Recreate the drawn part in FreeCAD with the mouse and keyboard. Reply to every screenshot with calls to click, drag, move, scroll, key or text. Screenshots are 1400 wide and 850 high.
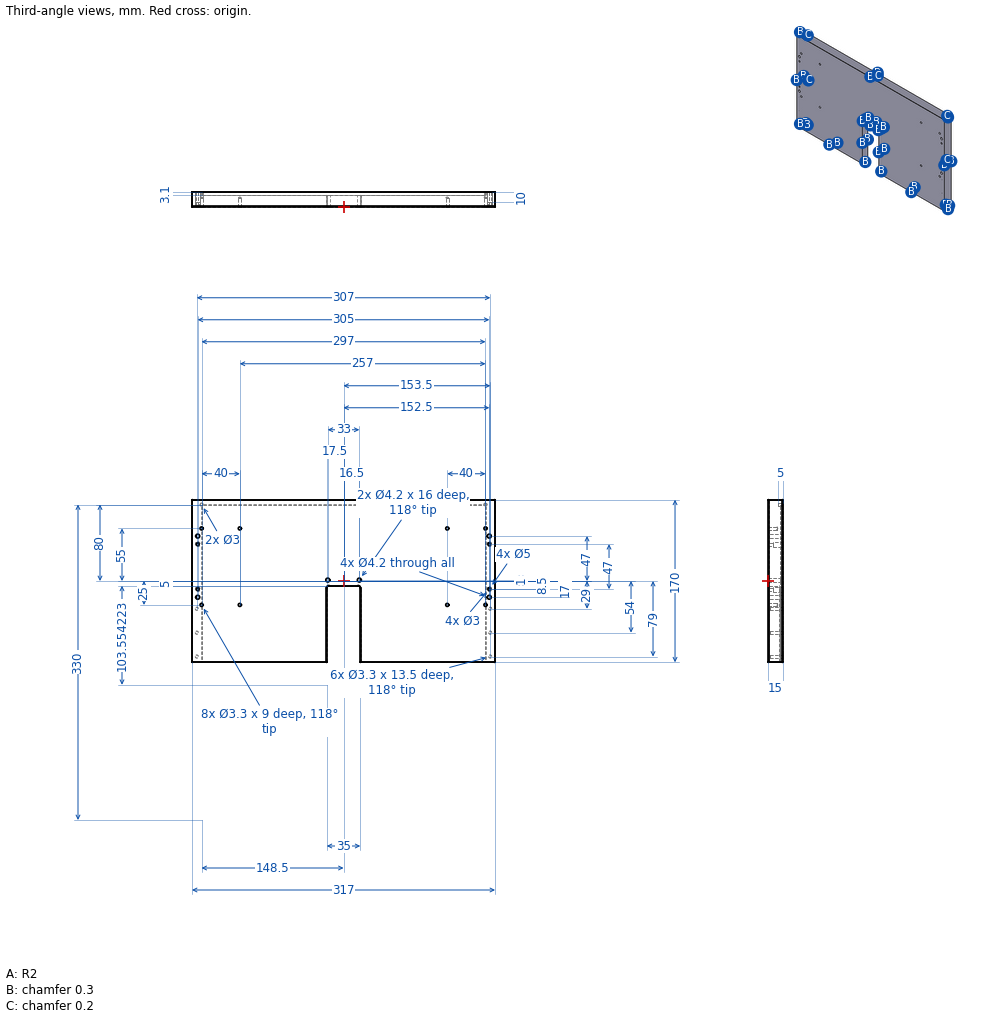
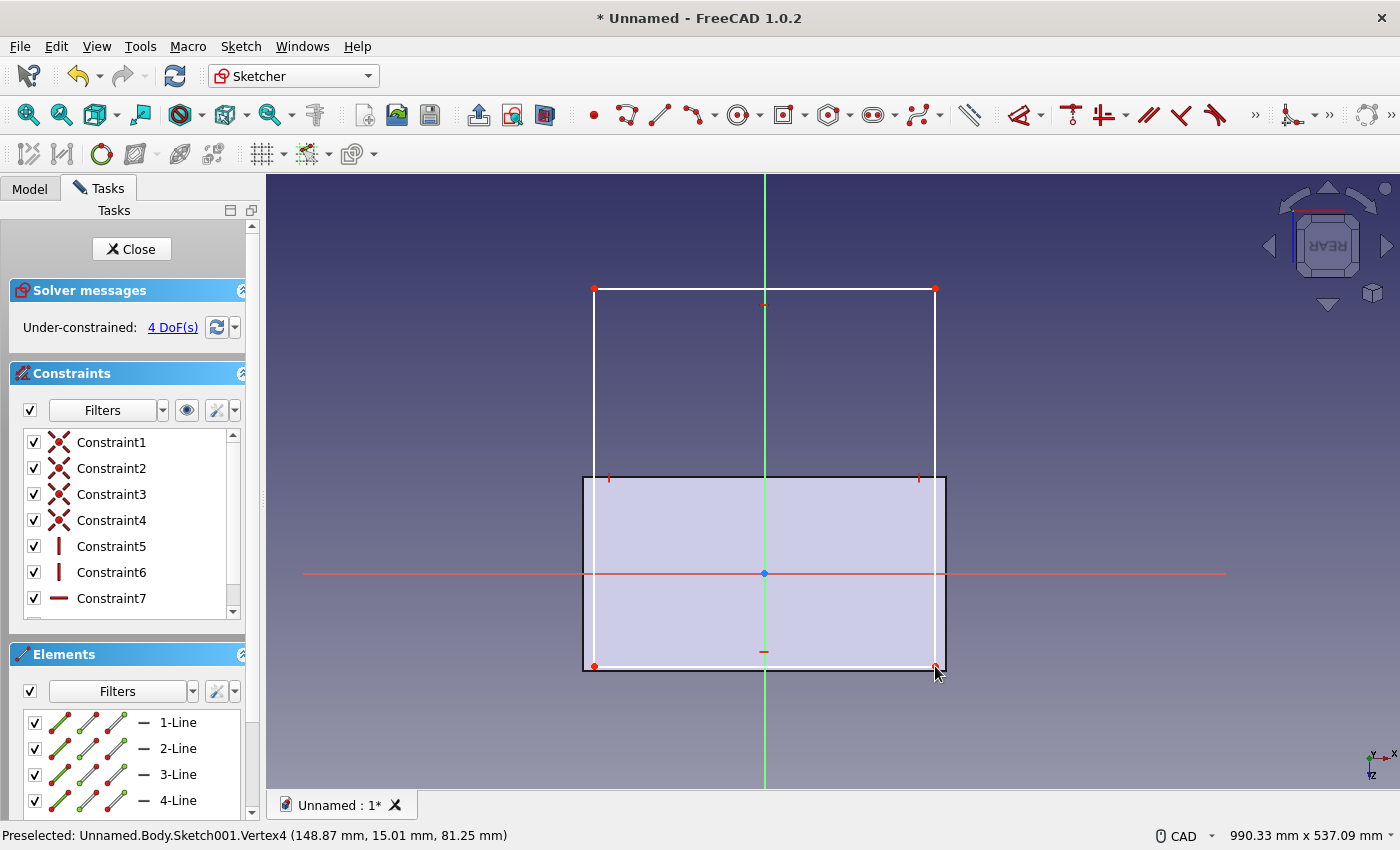
click(1018, 116)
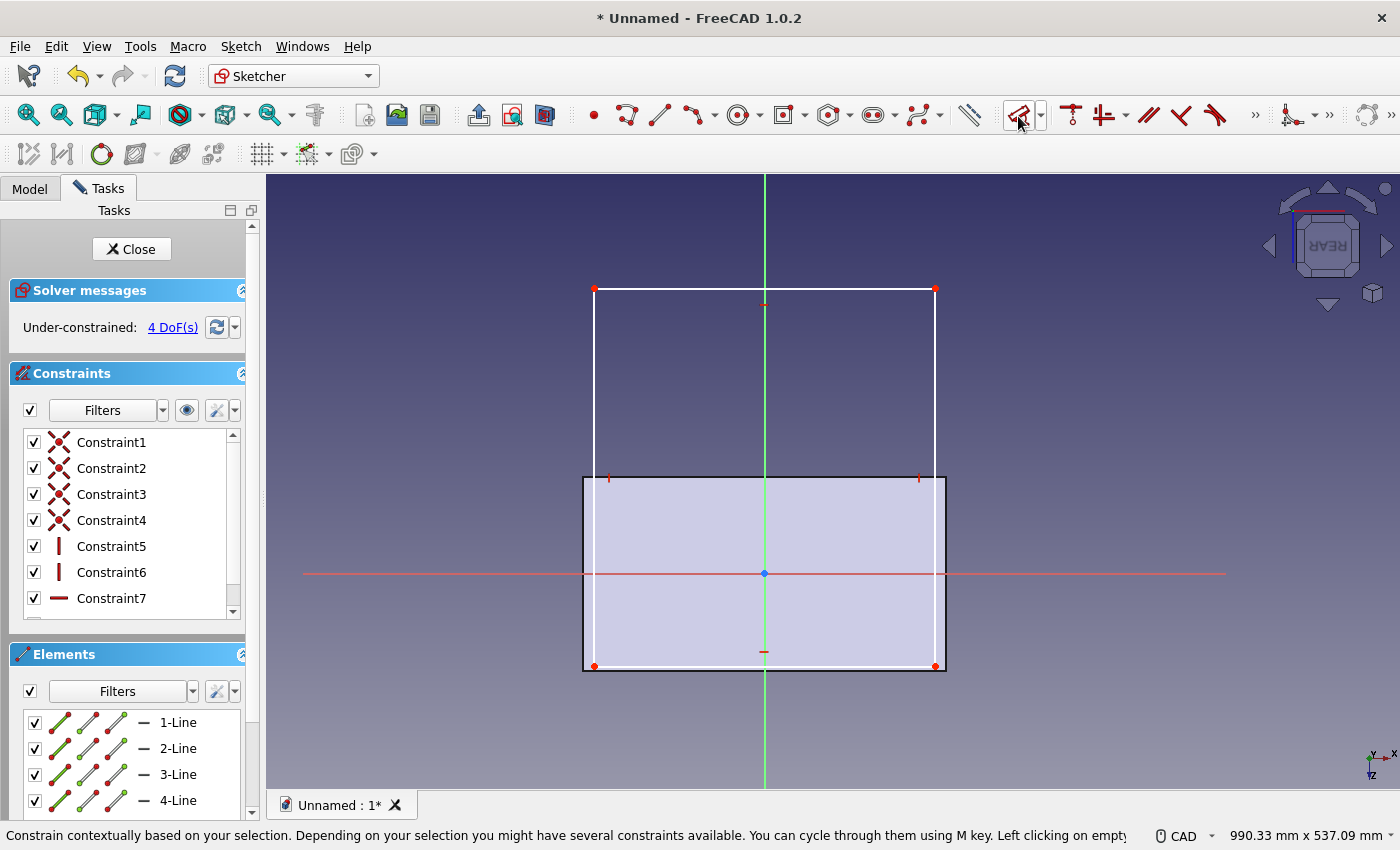
click(594, 402)
click(560, 478)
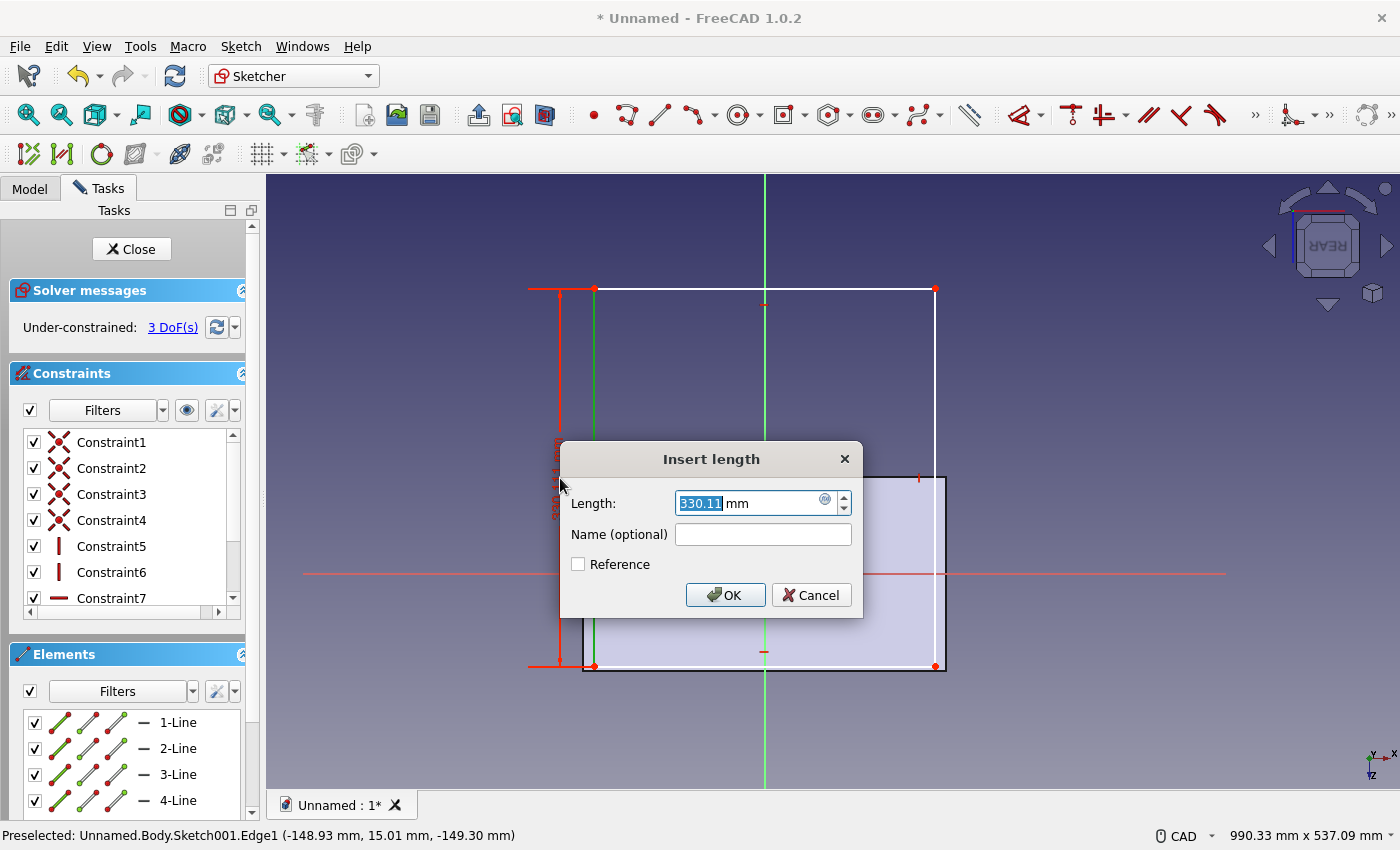
text(330)
key(Return)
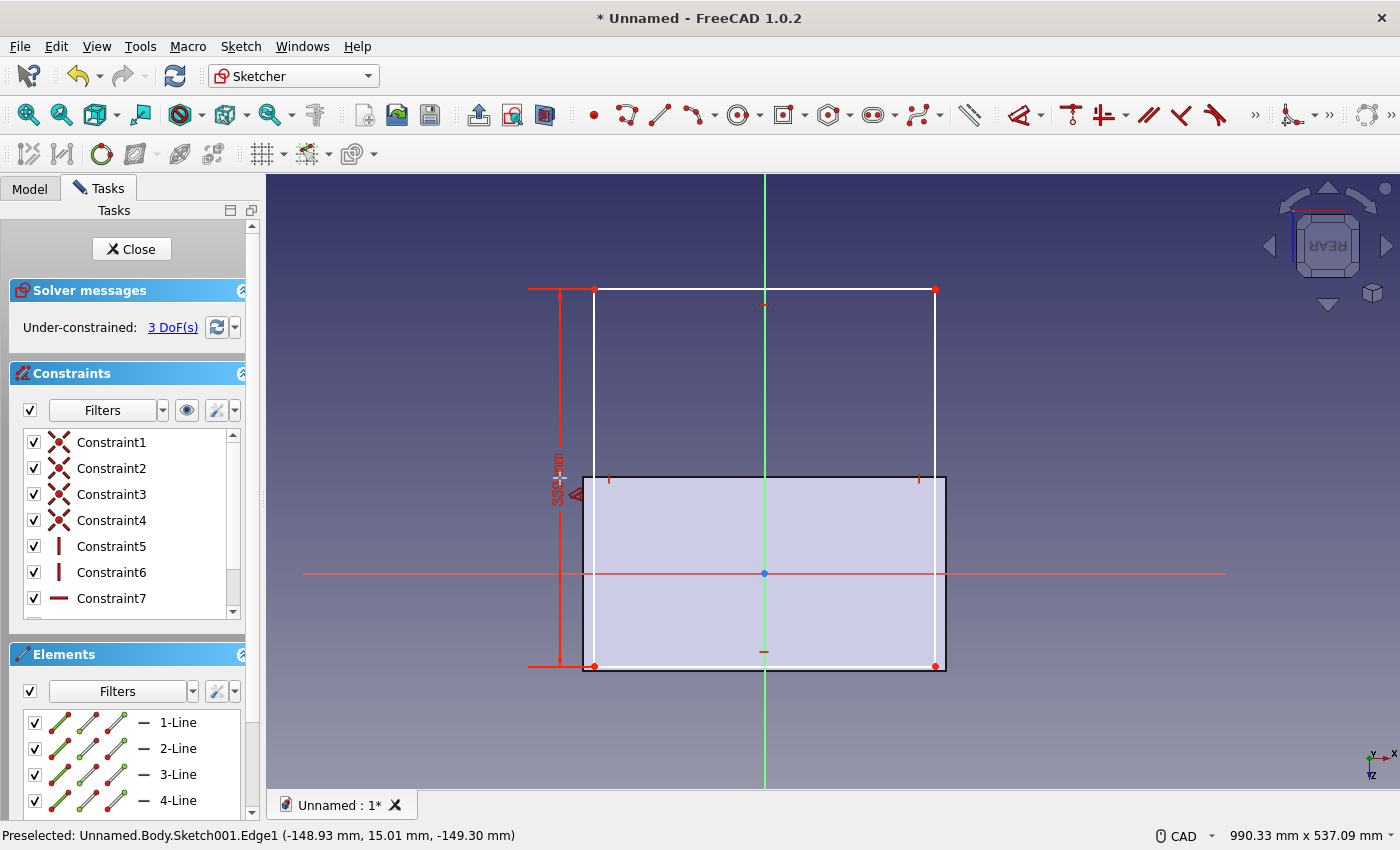
click(696, 667)
click(686, 701)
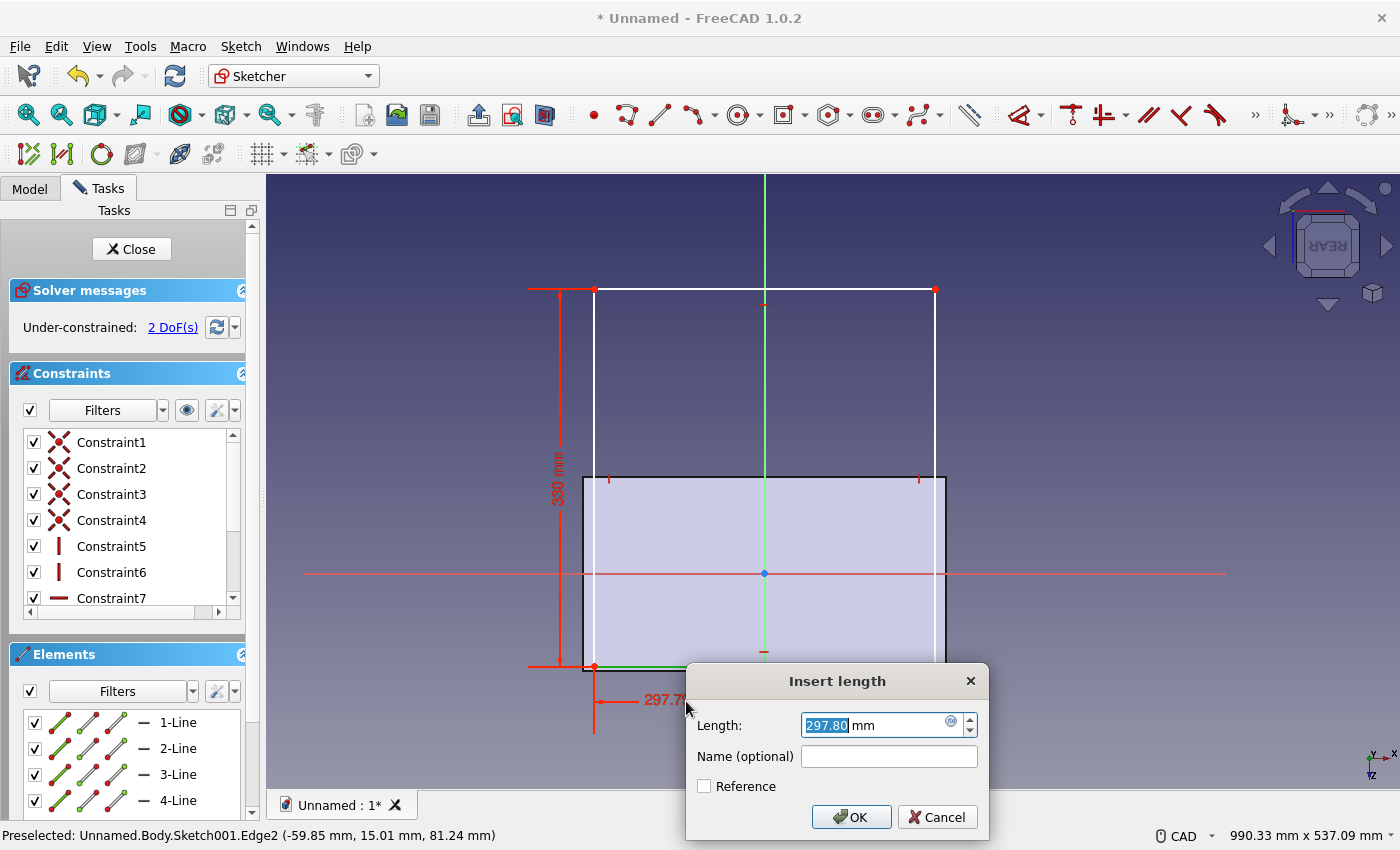
text(297)
key(Return)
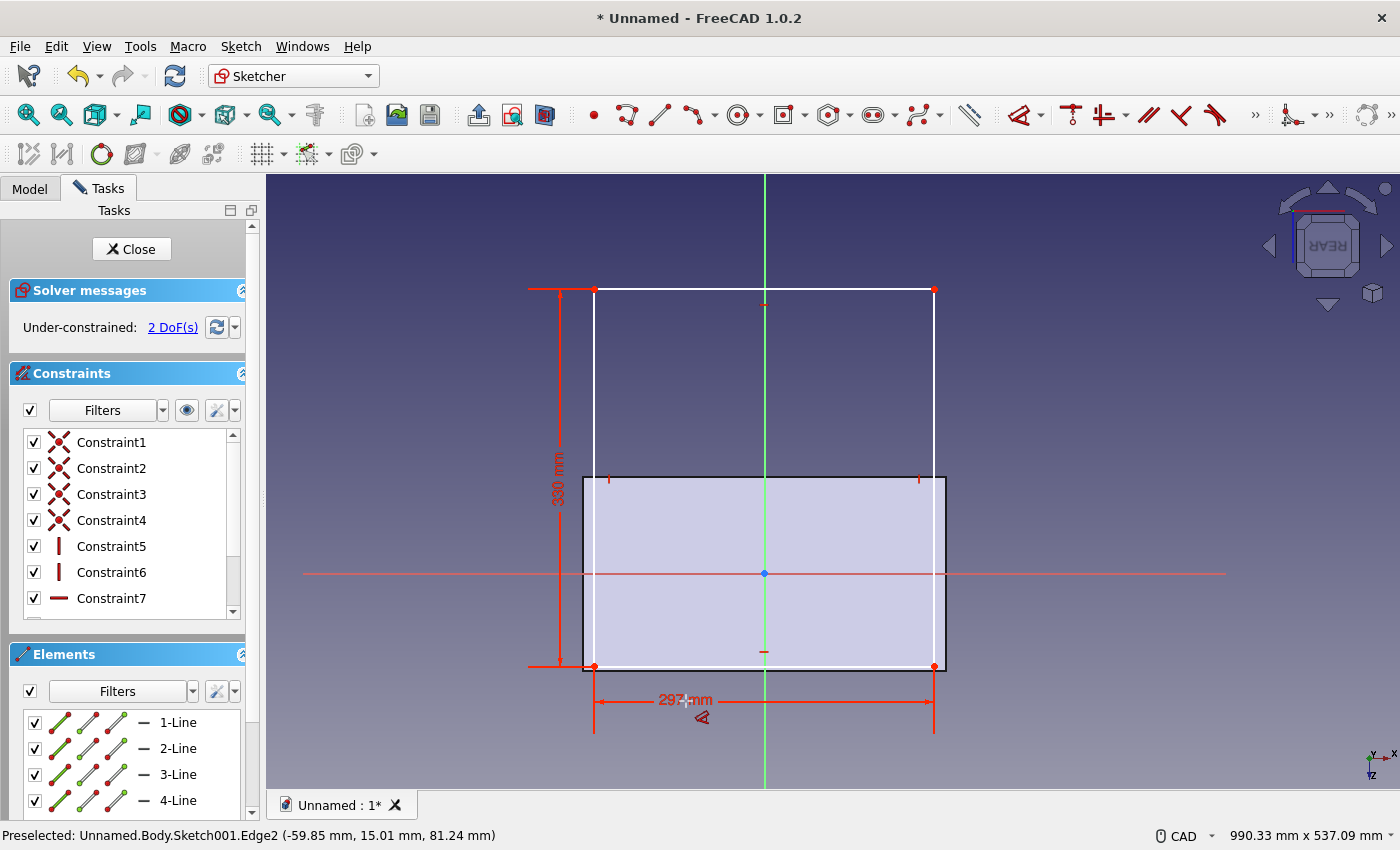
click(594, 667)
click(560, 620)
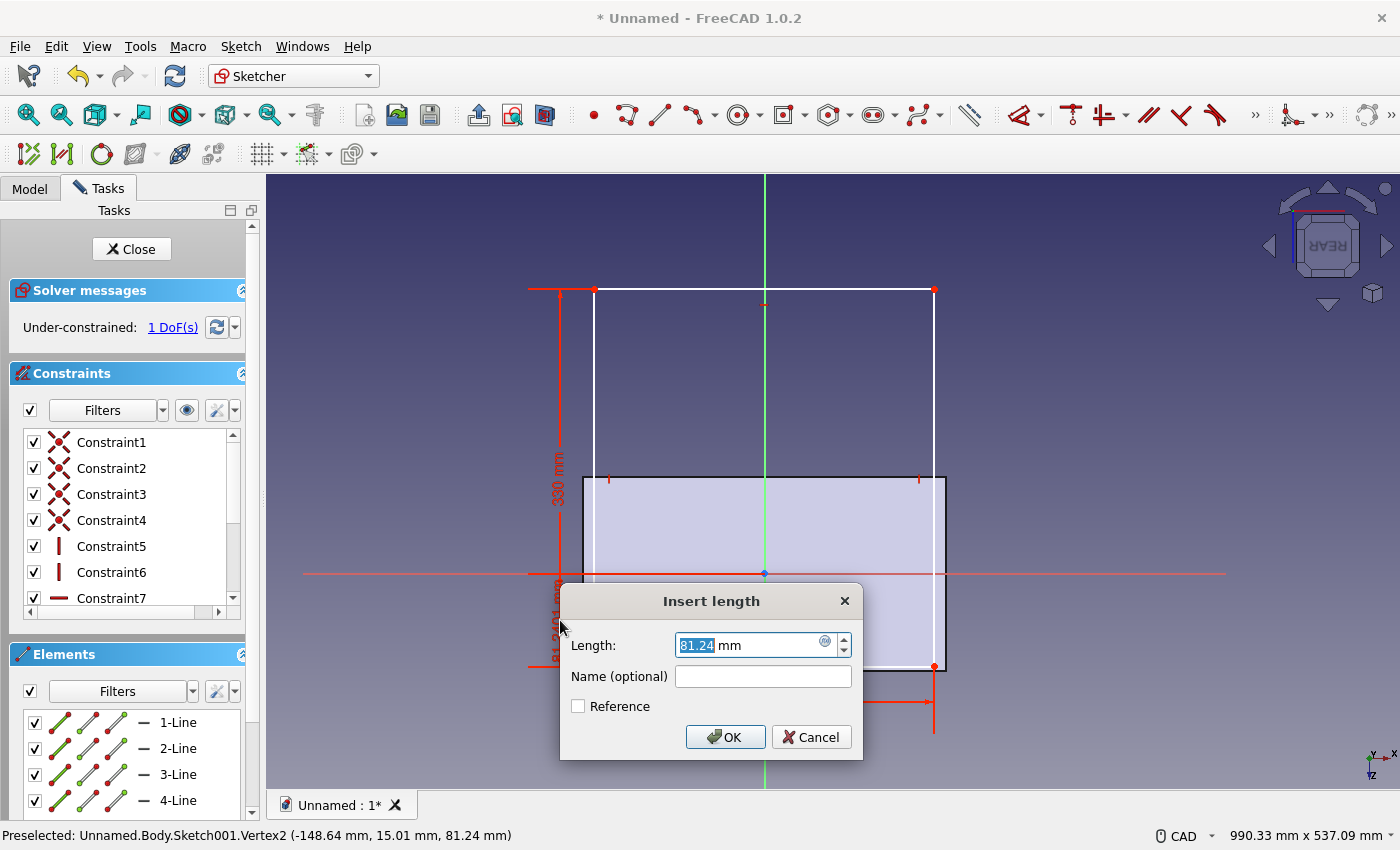
text(80)
key(Return)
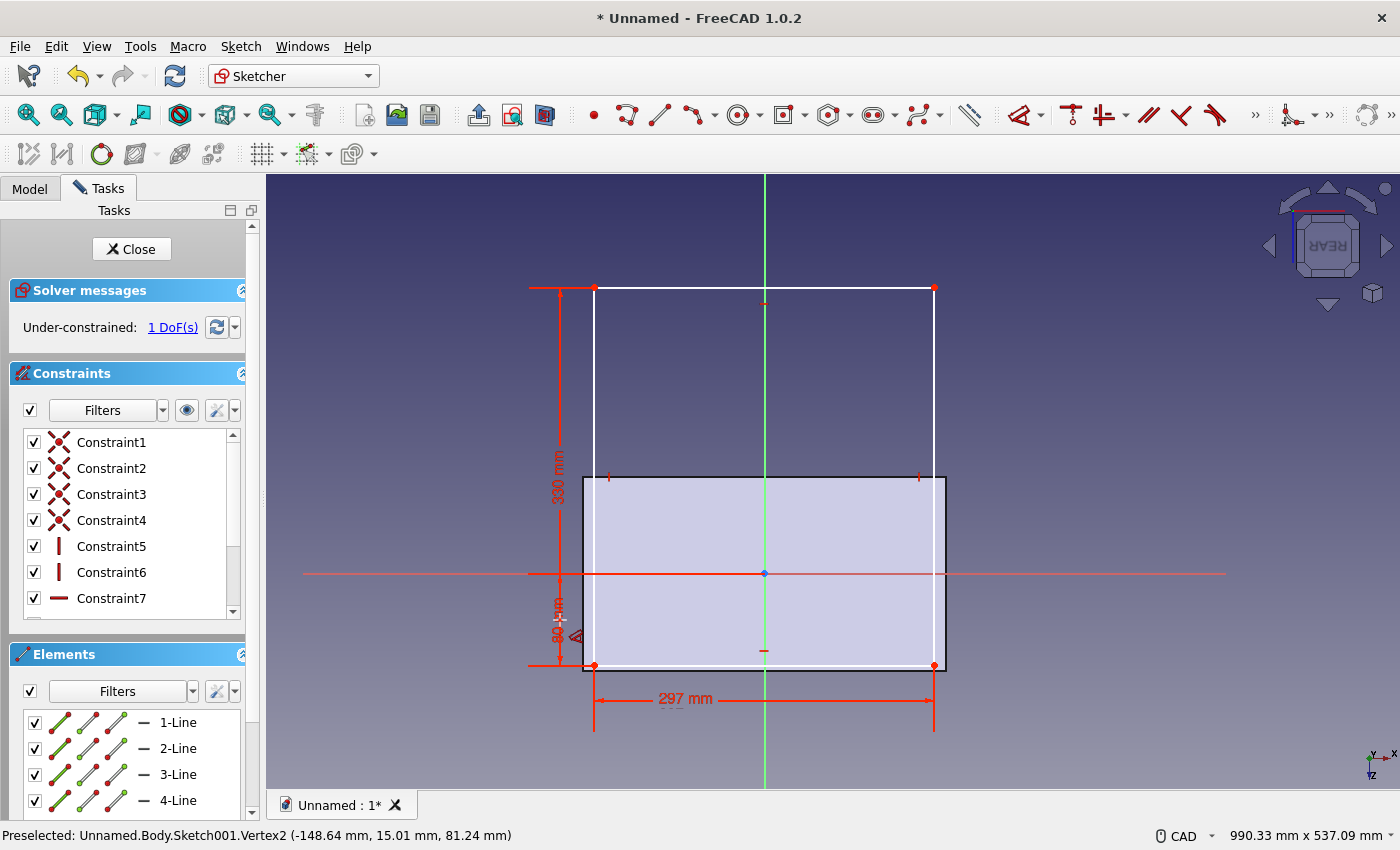
click(594, 288)
click(679, 254)